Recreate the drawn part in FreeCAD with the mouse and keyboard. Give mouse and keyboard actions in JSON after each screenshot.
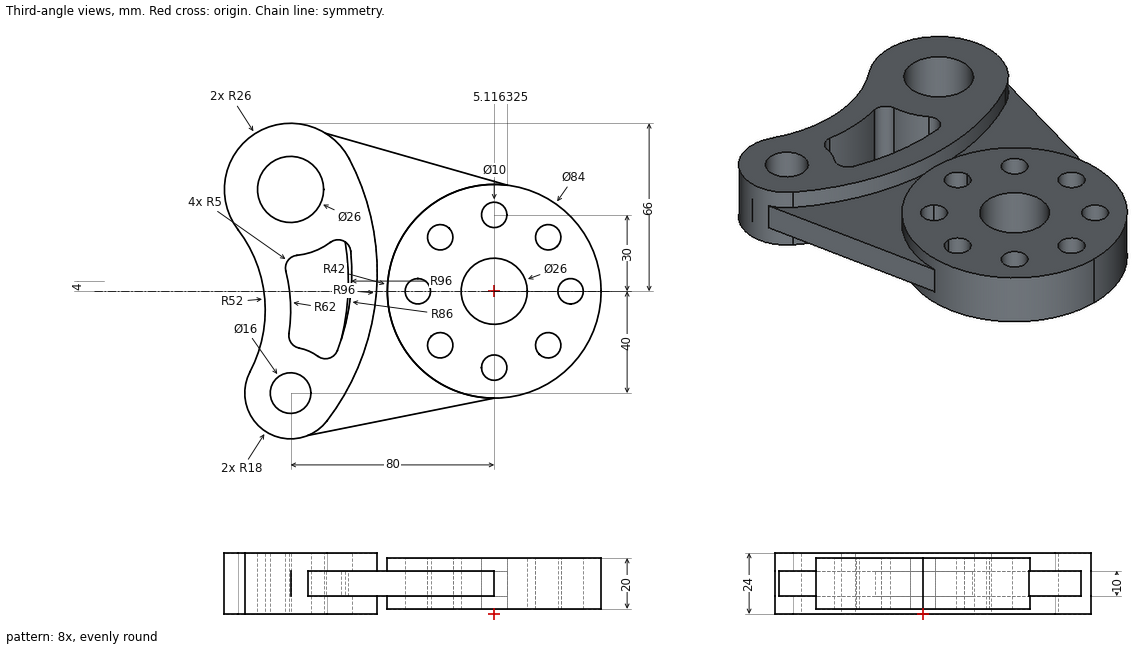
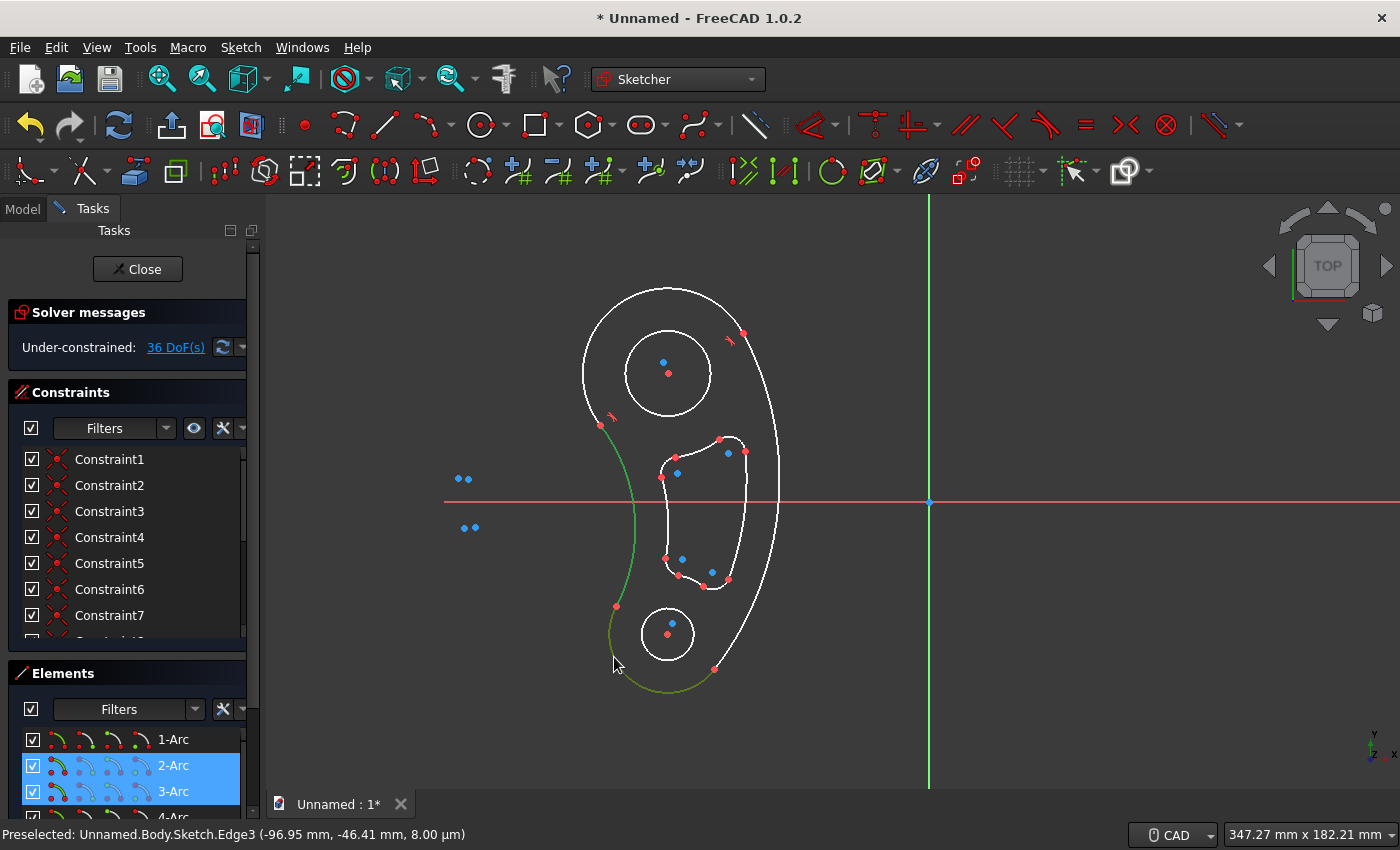
{"action": "left_click", "coordinate": [1046, 126]}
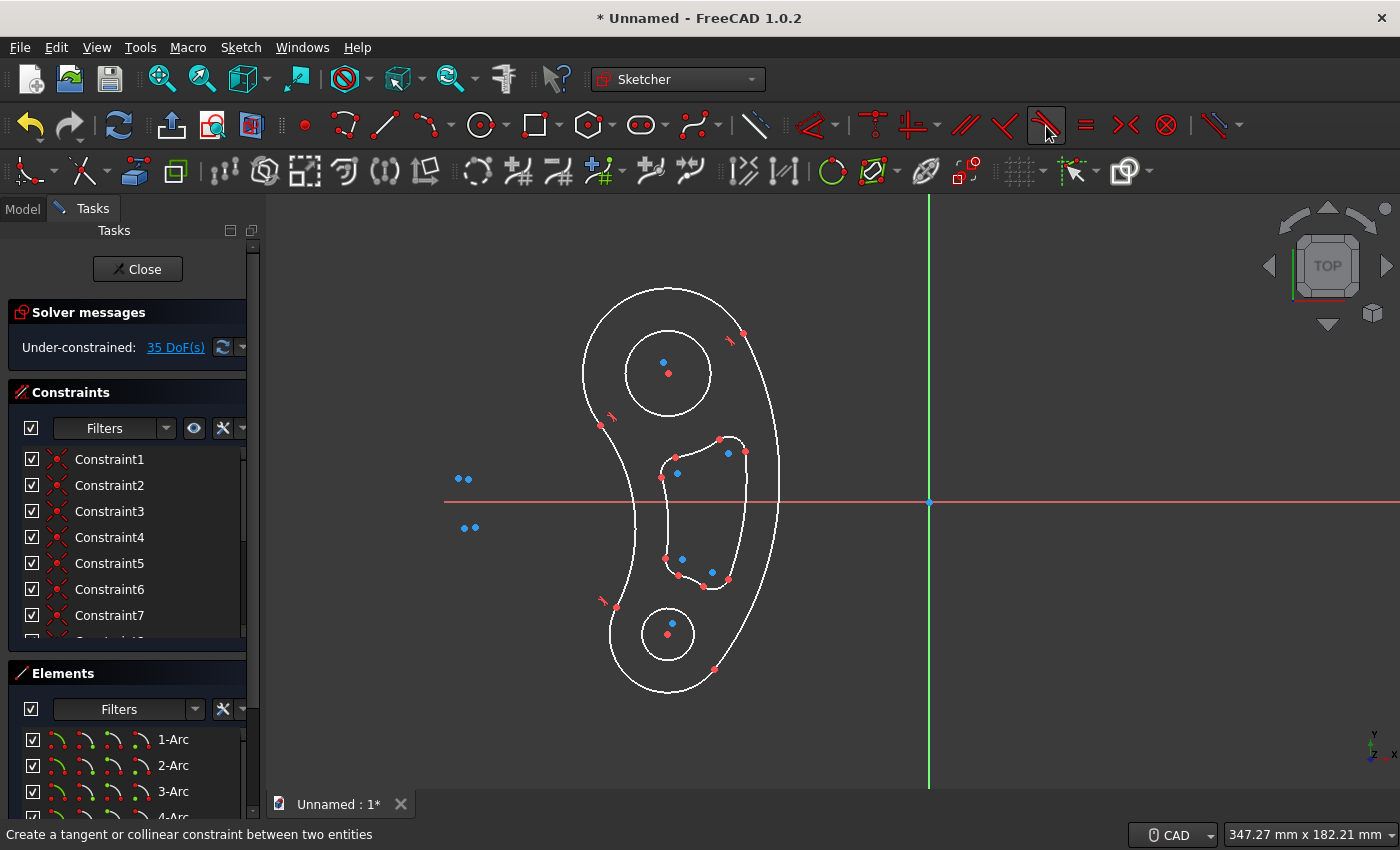
{"action": "left_click", "coordinate": [615, 658]}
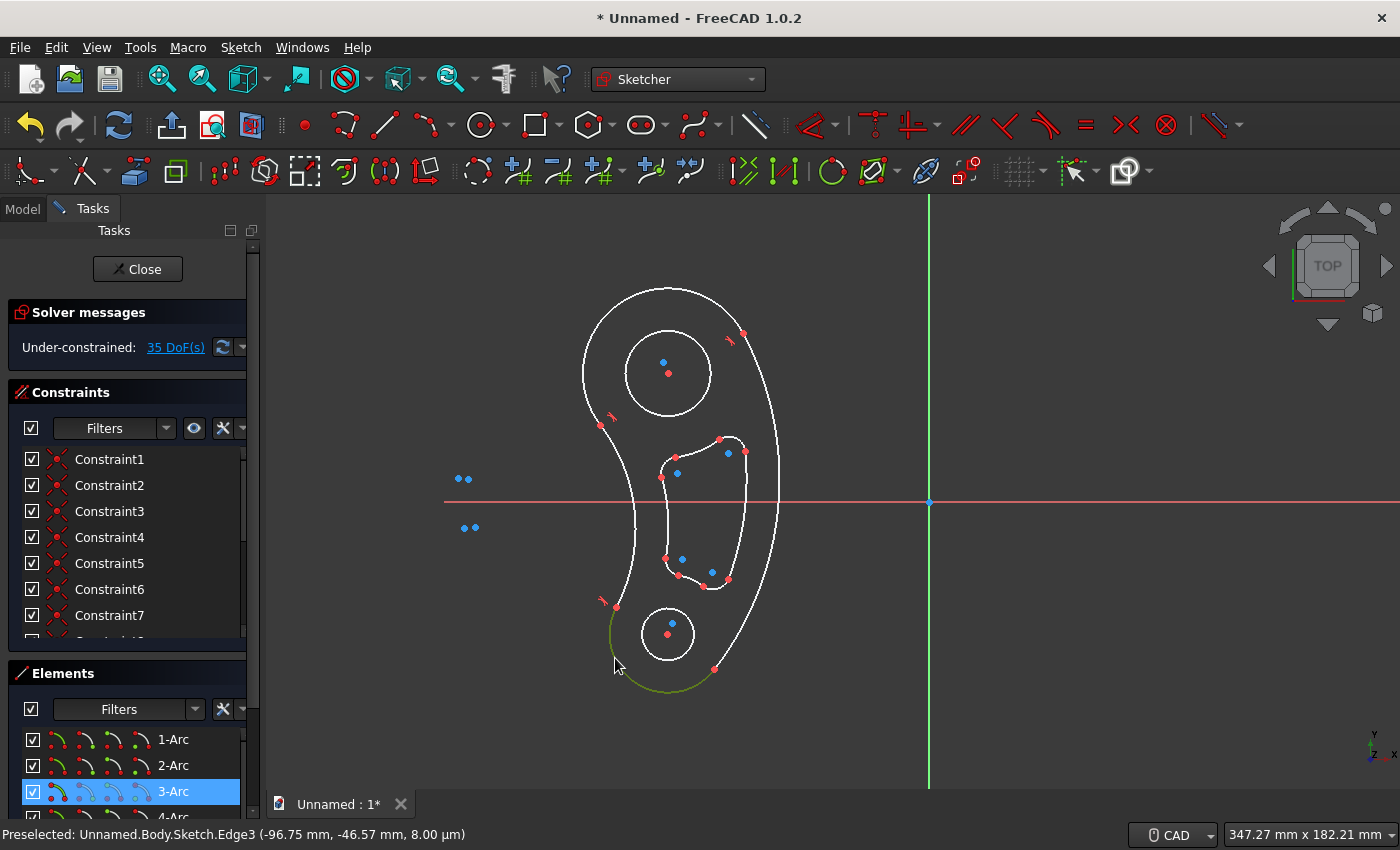
{"action": "left_click", "coordinate": [764, 576]}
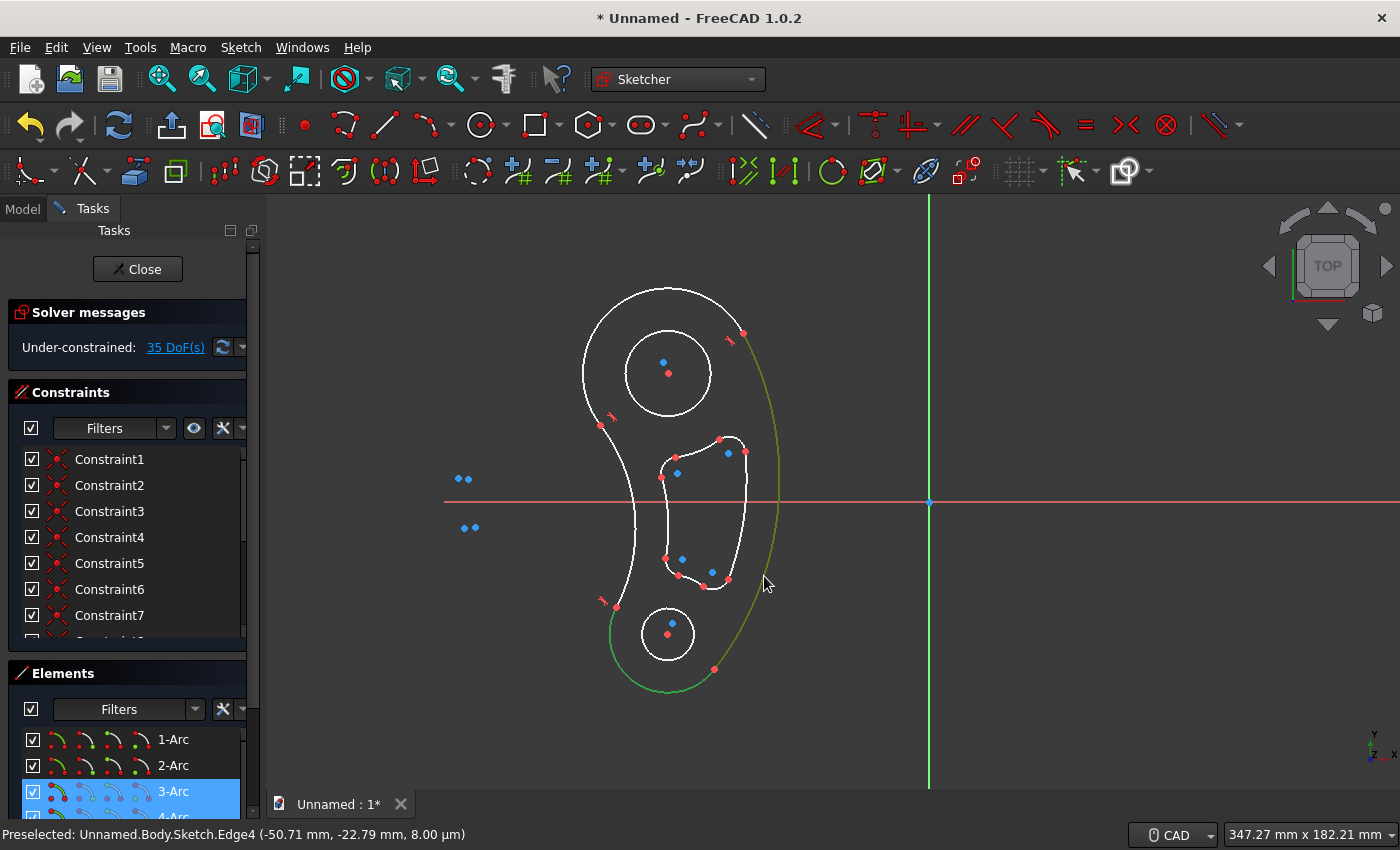
{"action": "left_click", "coordinate": [1046, 126]}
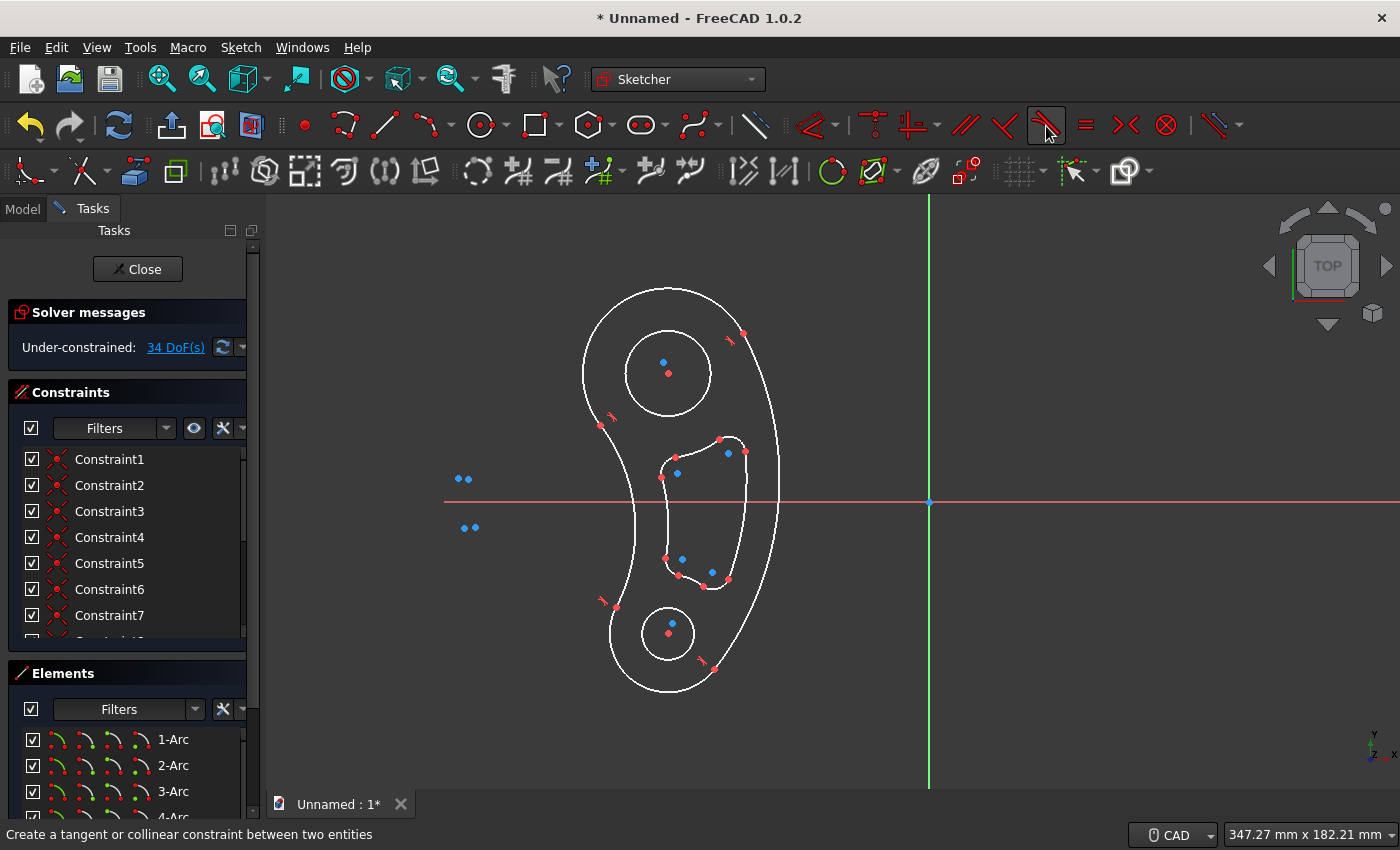
{"action": "left_click", "coordinate": [739, 542]}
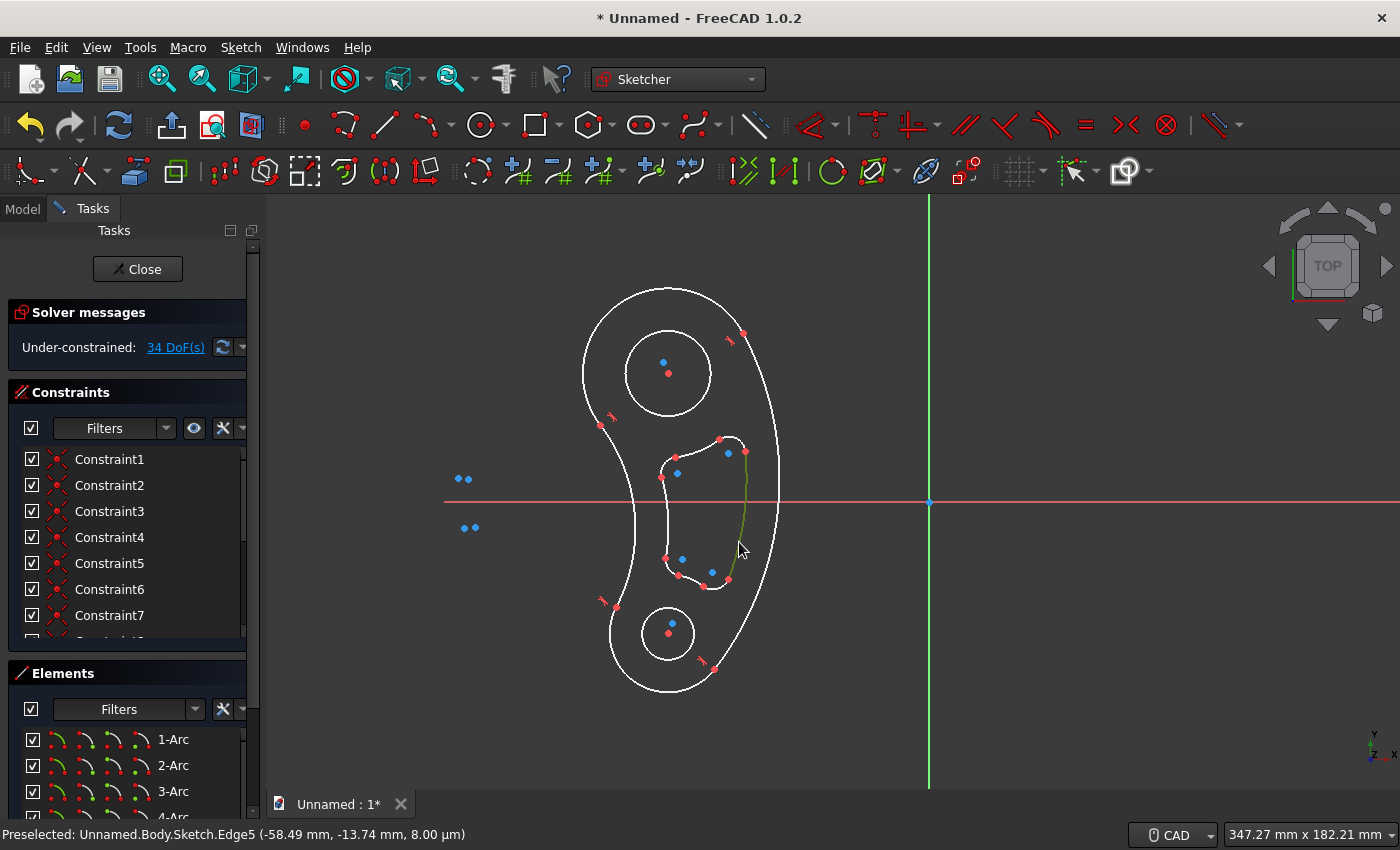
{"action": "left_click", "coordinate": [717, 589]}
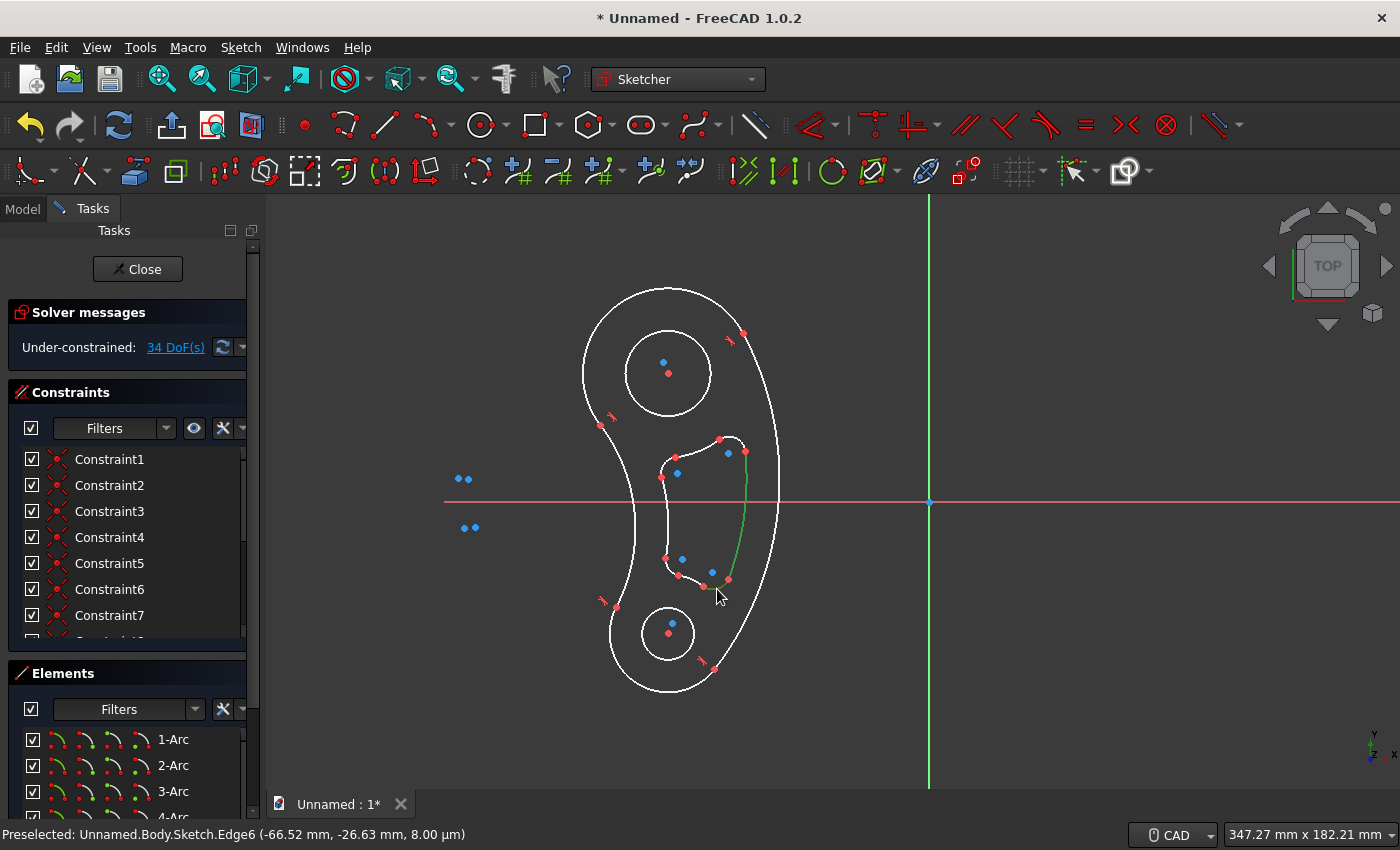
{"action": "left_click", "coordinate": [1046, 126]}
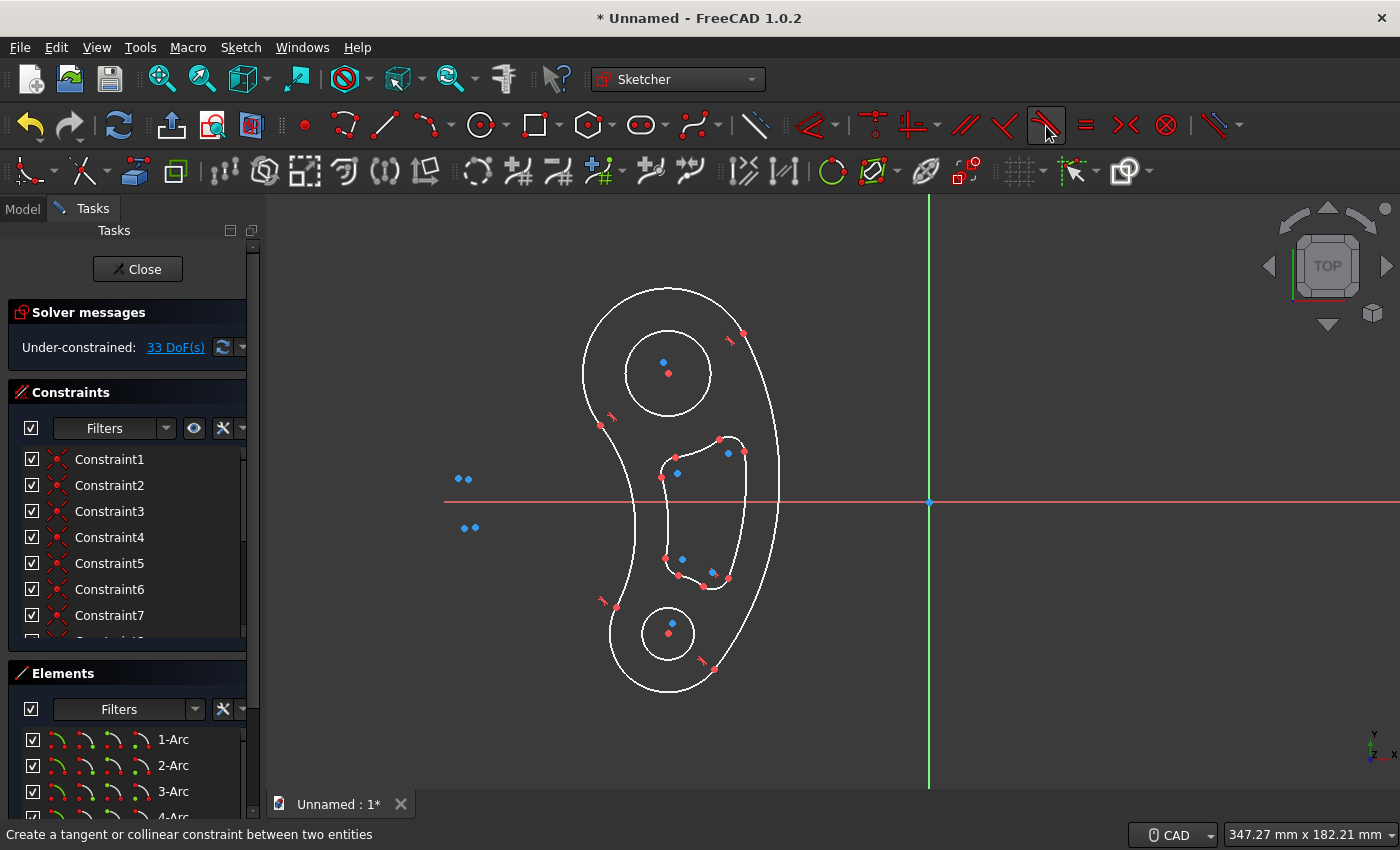
{"action": "left_click", "coordinate": [739, 541]}